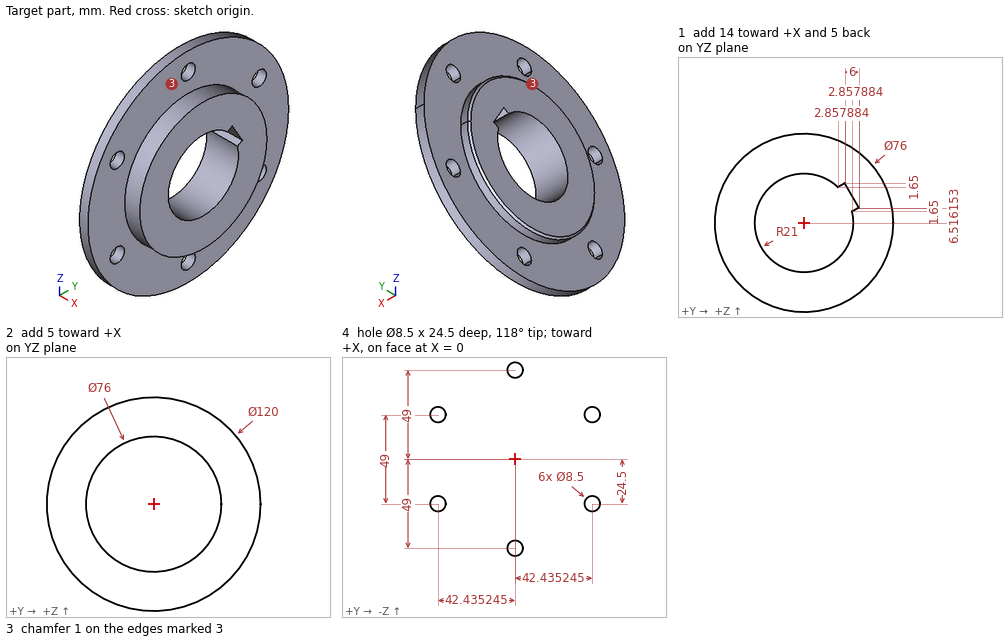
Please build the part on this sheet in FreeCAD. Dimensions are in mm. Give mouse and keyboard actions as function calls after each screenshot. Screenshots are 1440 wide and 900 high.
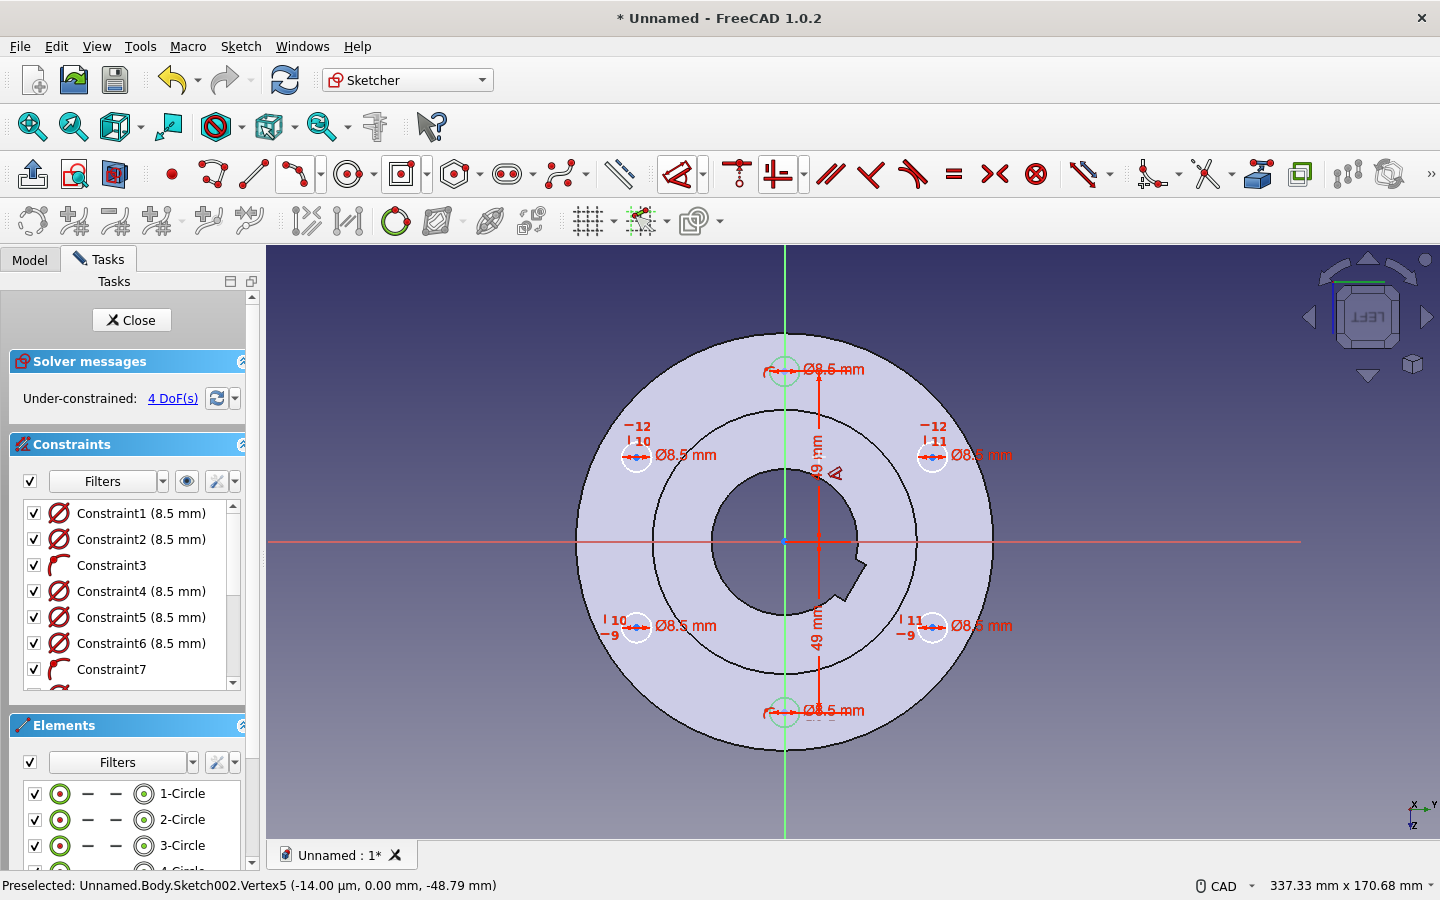
click(637, 628)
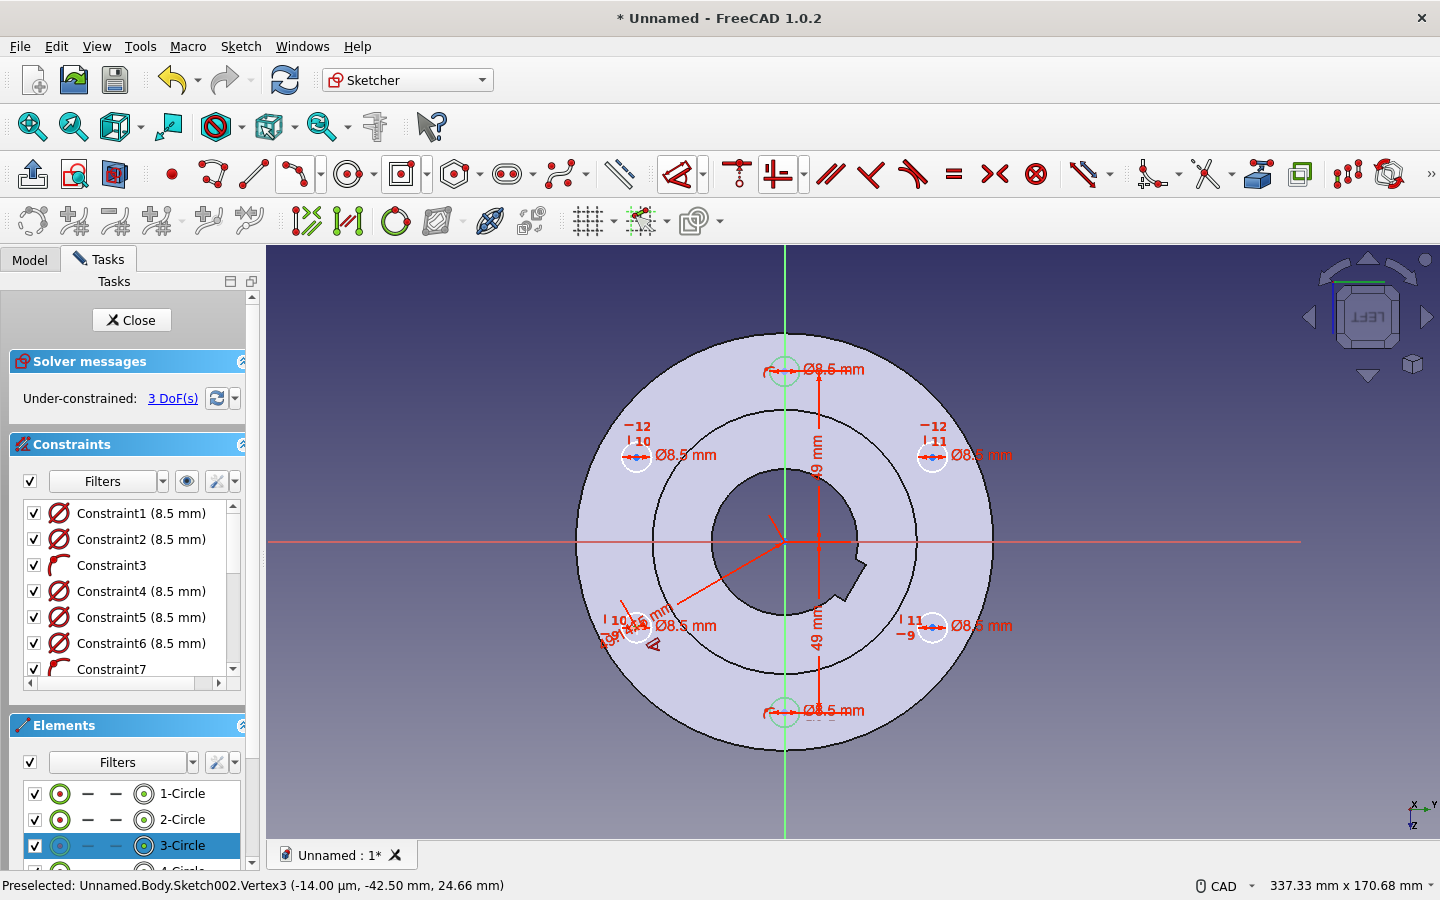
click(637, 457)
click(603, 503)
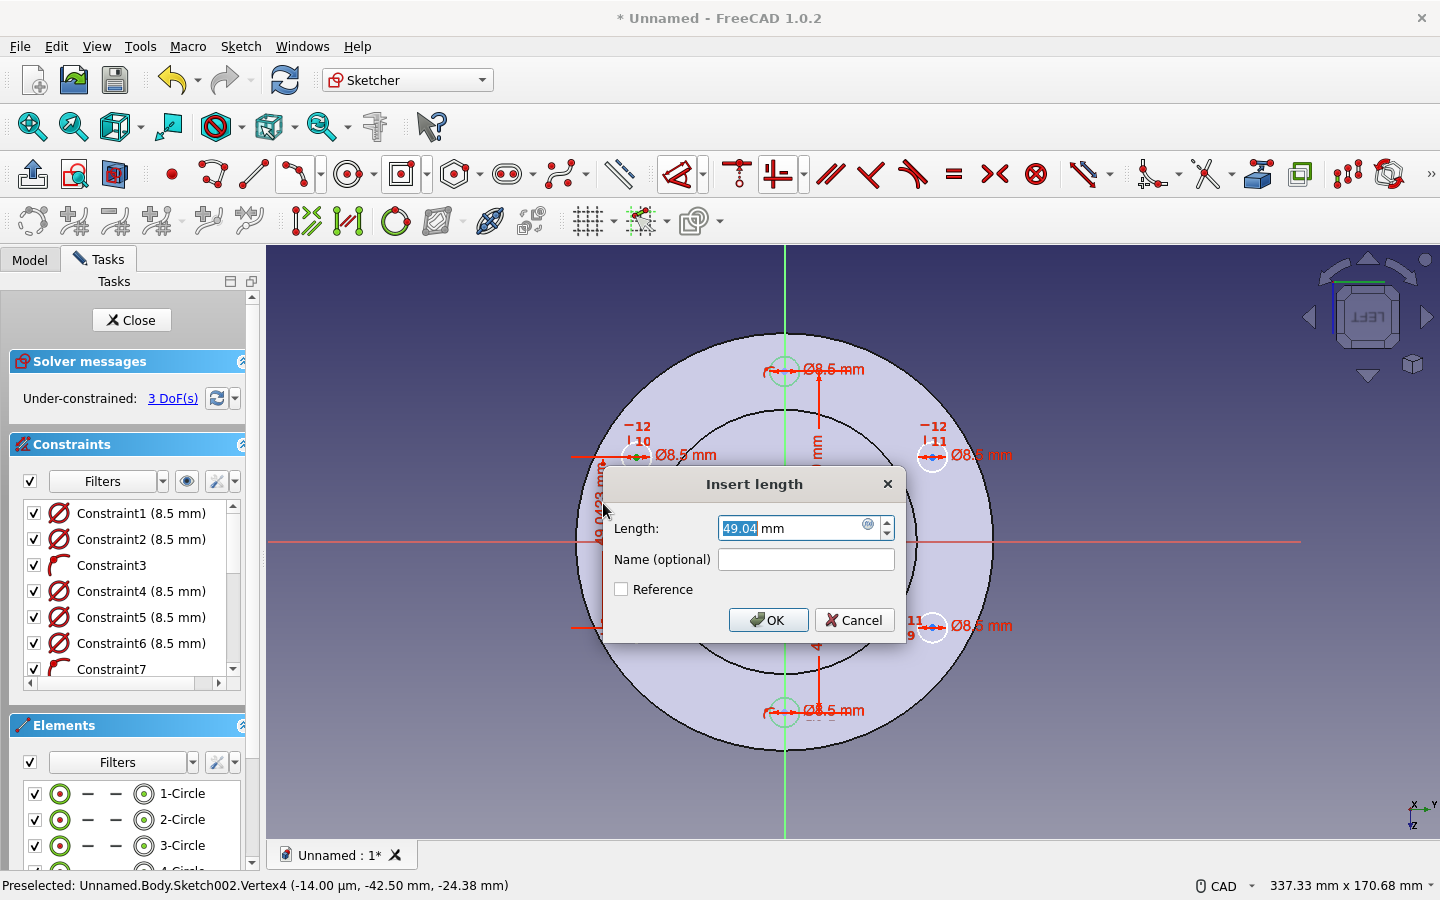
text(49)
key(Return)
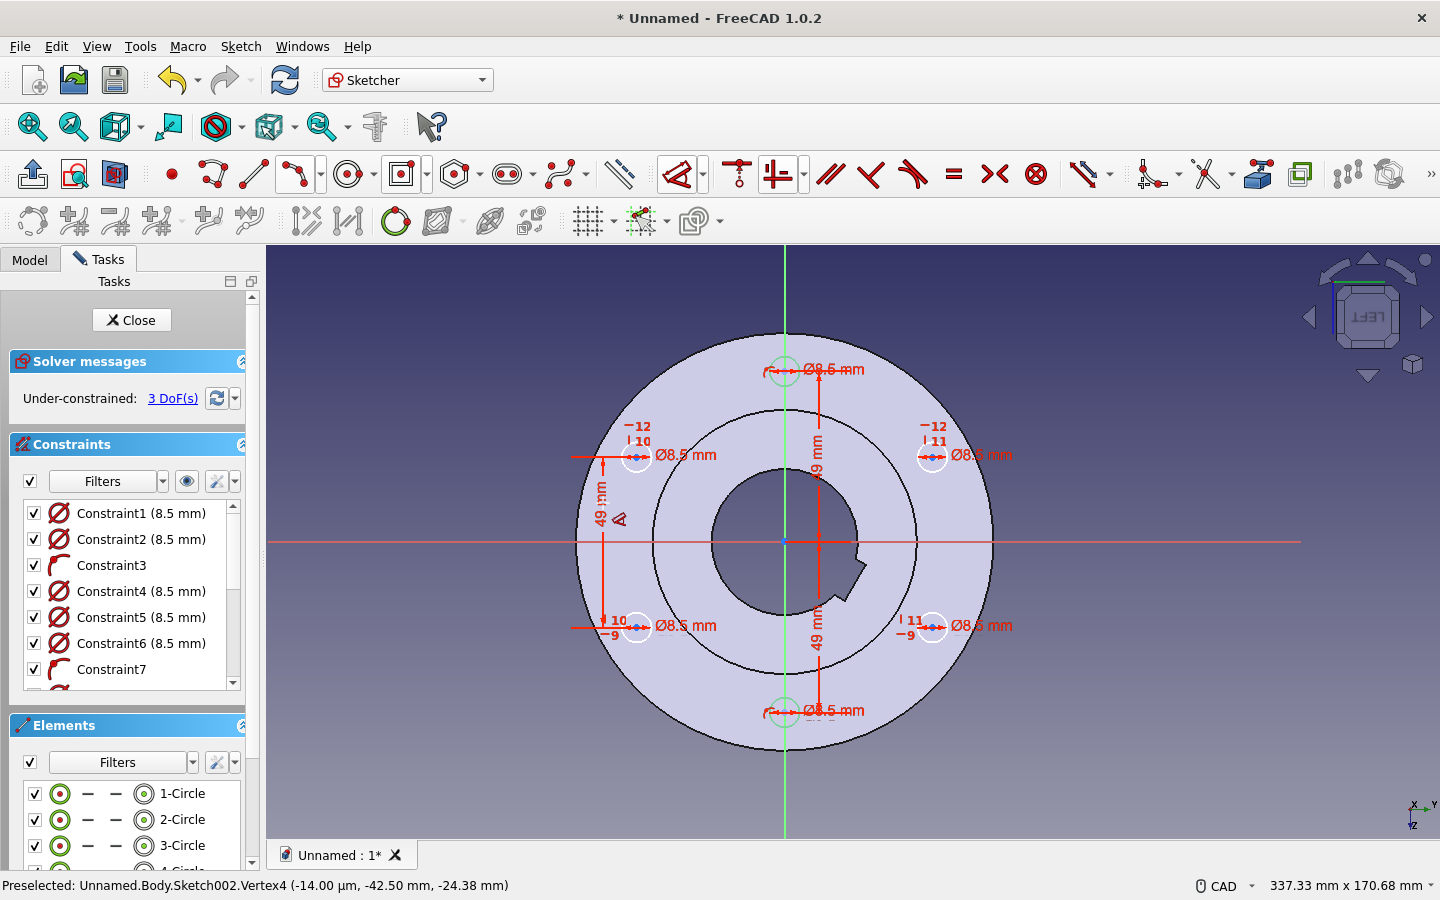
click(933, 628)
click(967, 585)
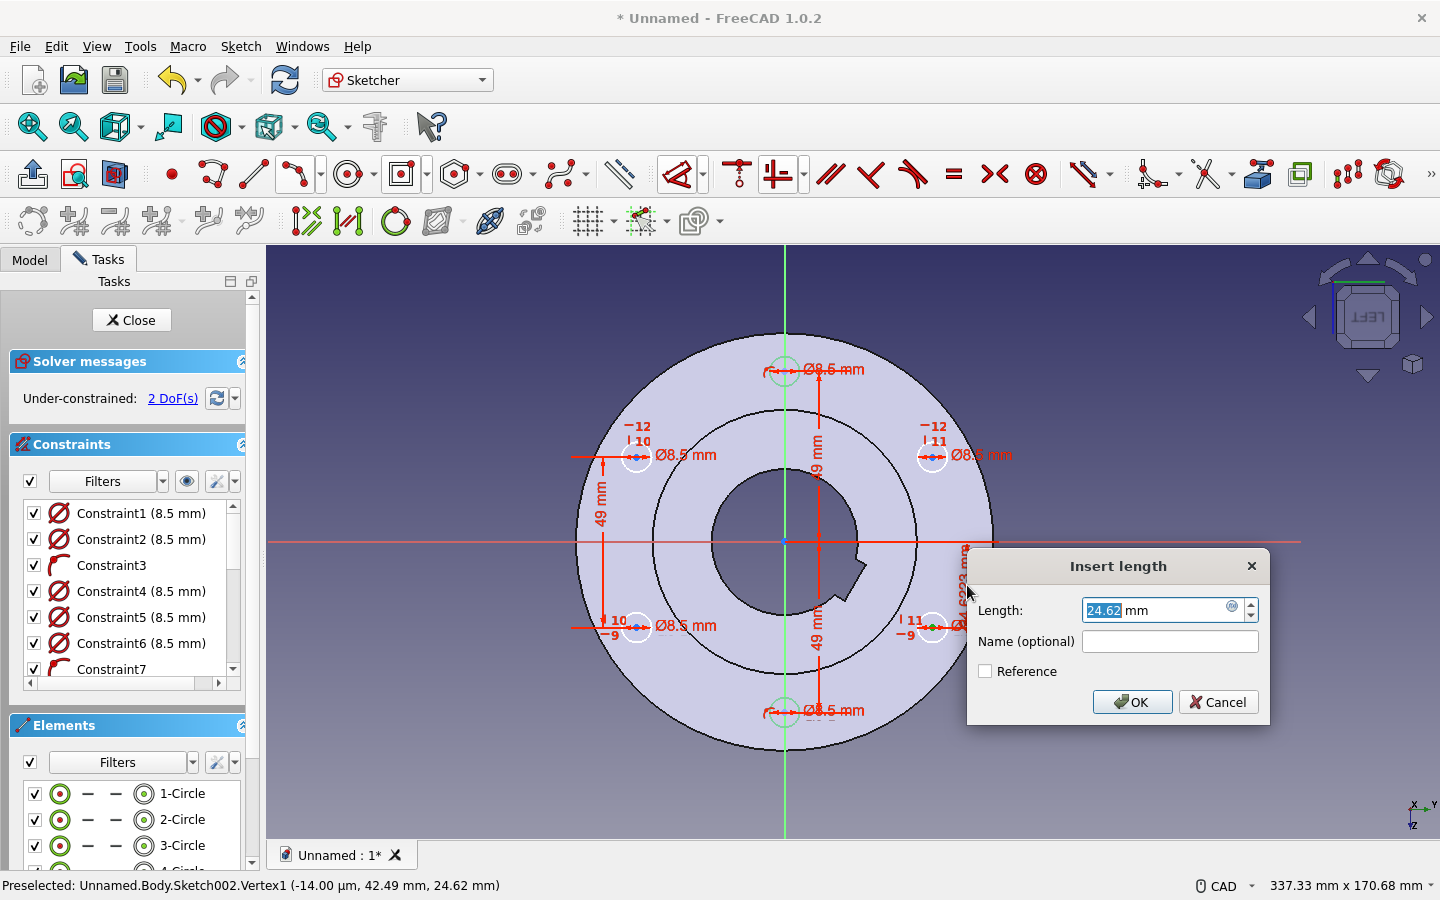
text(24.5)
key(Return)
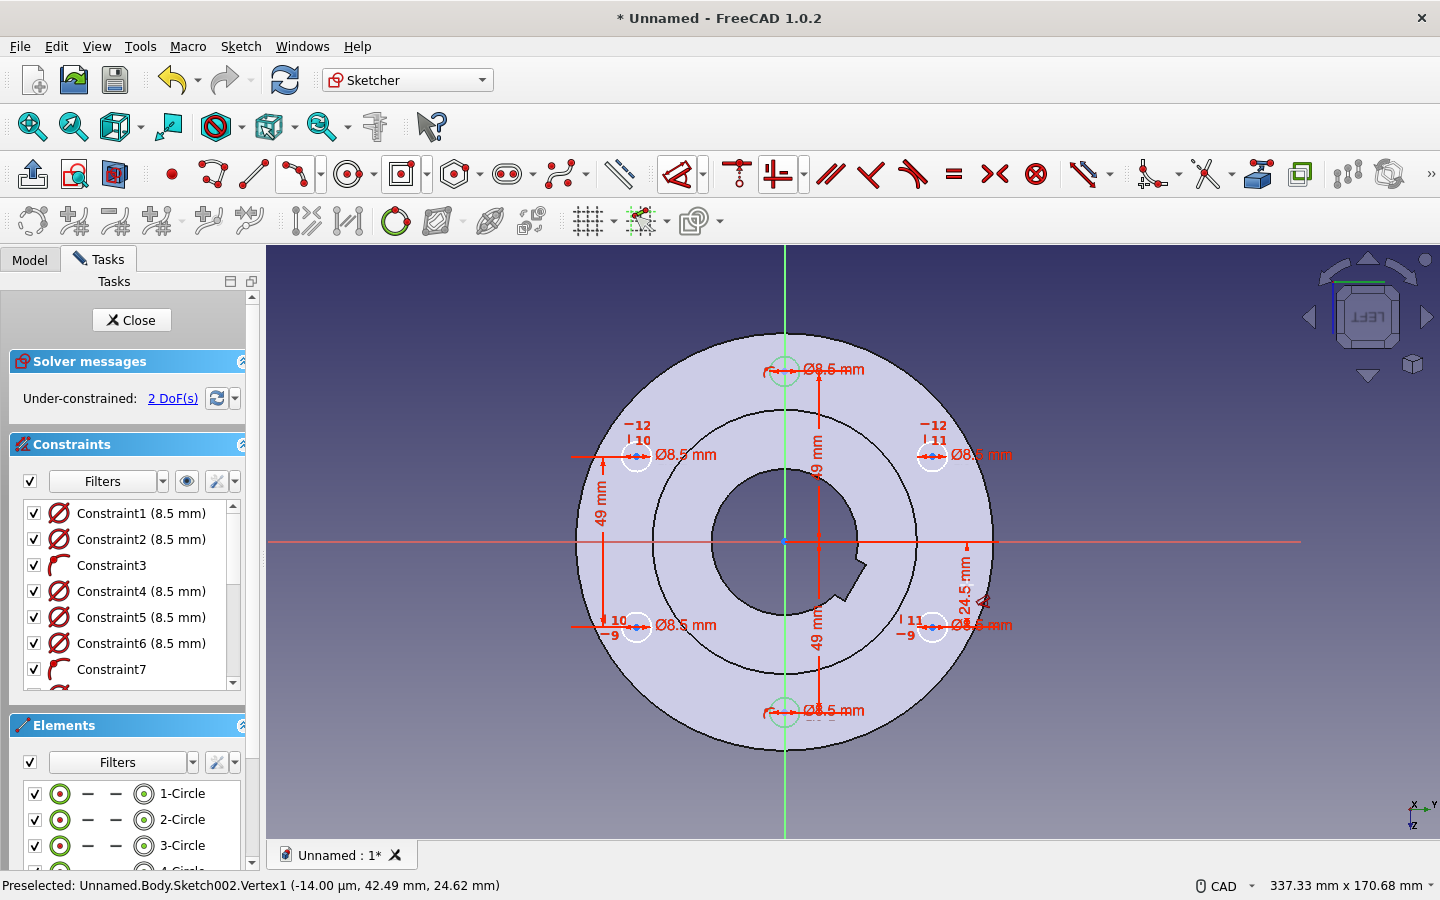
click(933, 627)
click(859, 661)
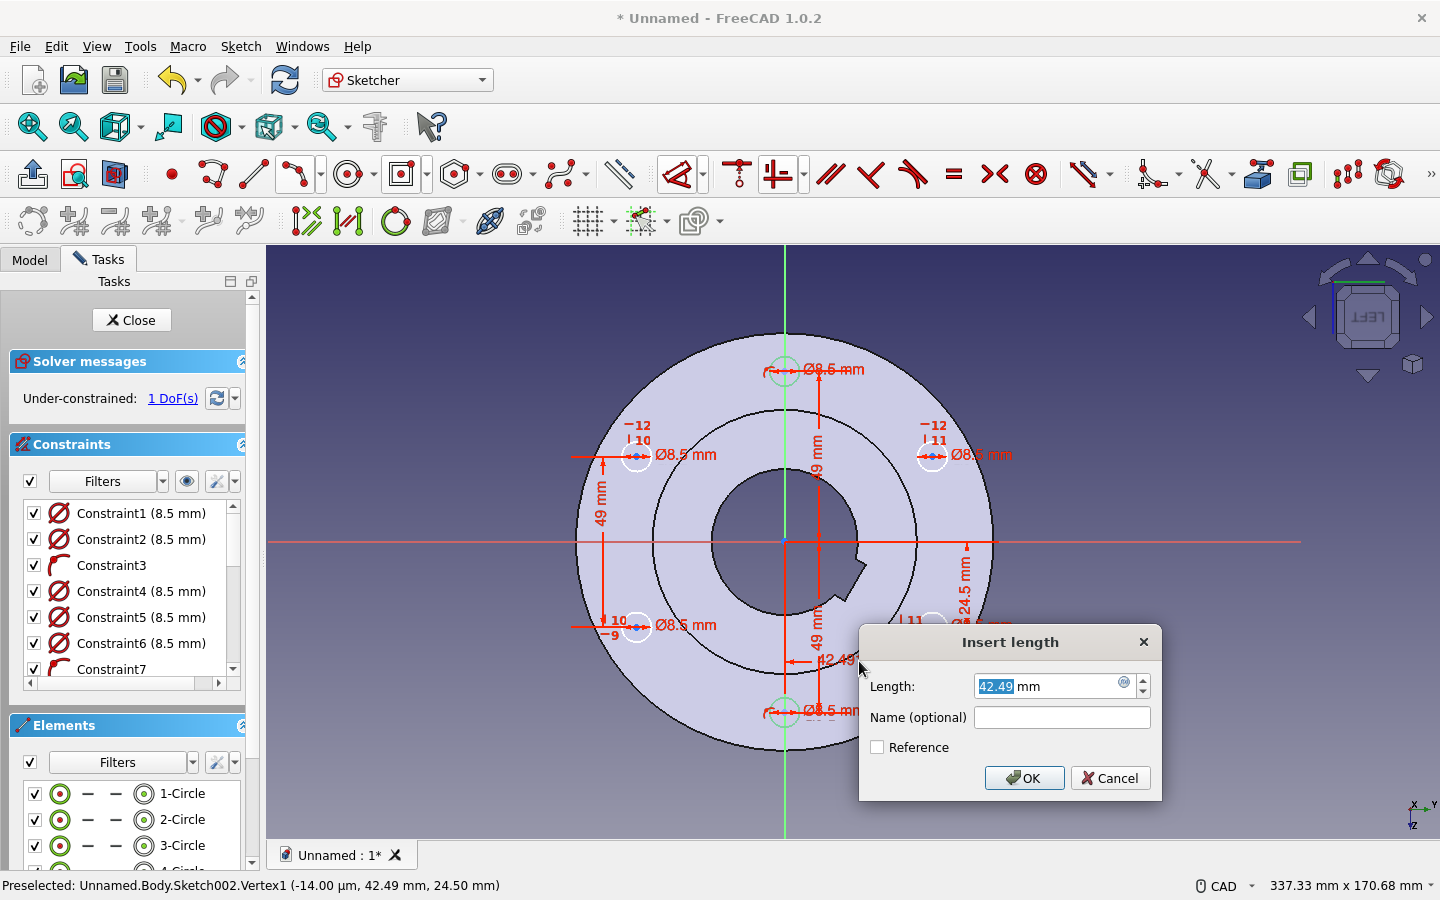
text(42.435245)
key(Return)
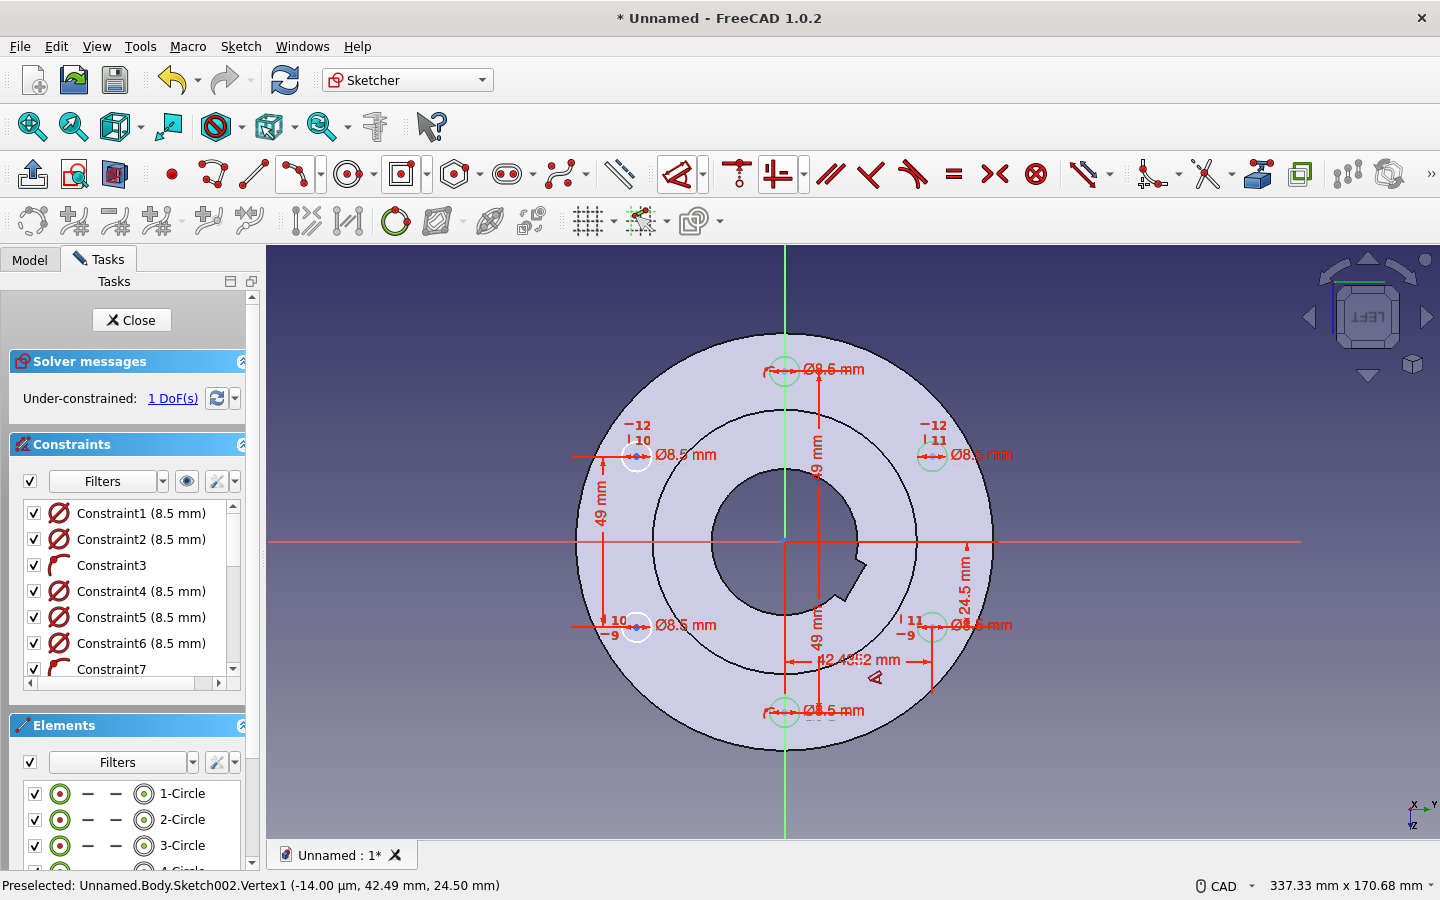
click(637, 627)
click(711, 661)